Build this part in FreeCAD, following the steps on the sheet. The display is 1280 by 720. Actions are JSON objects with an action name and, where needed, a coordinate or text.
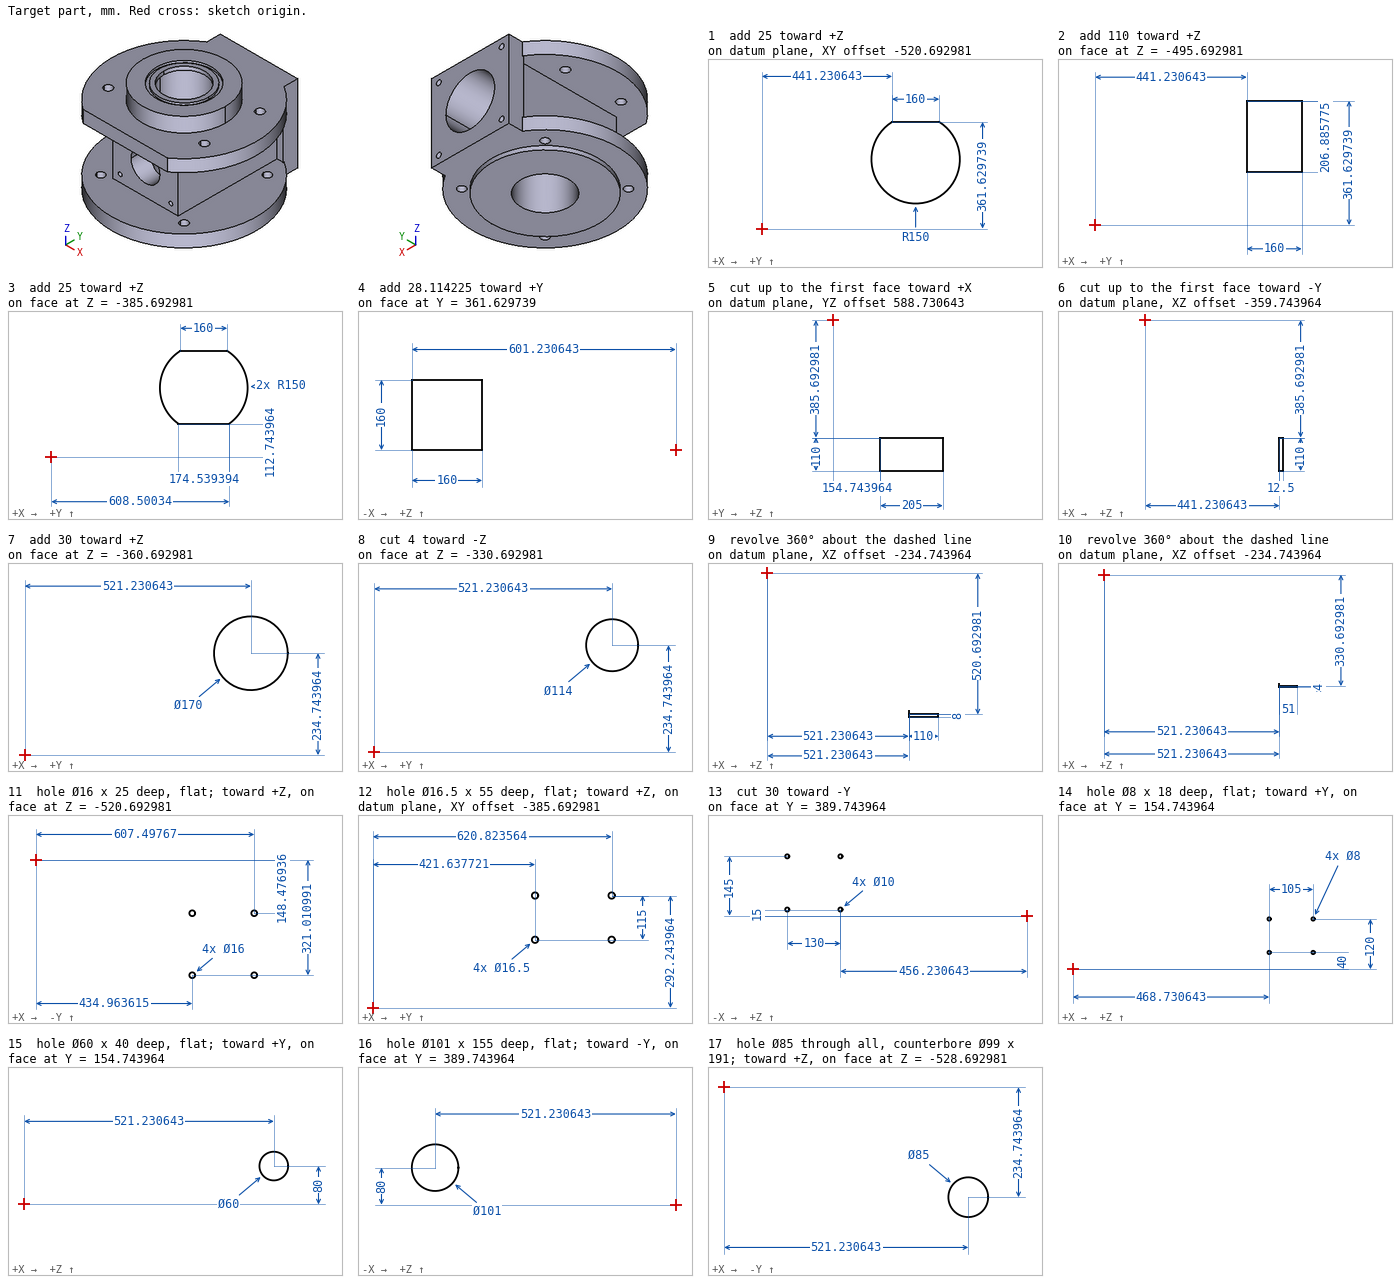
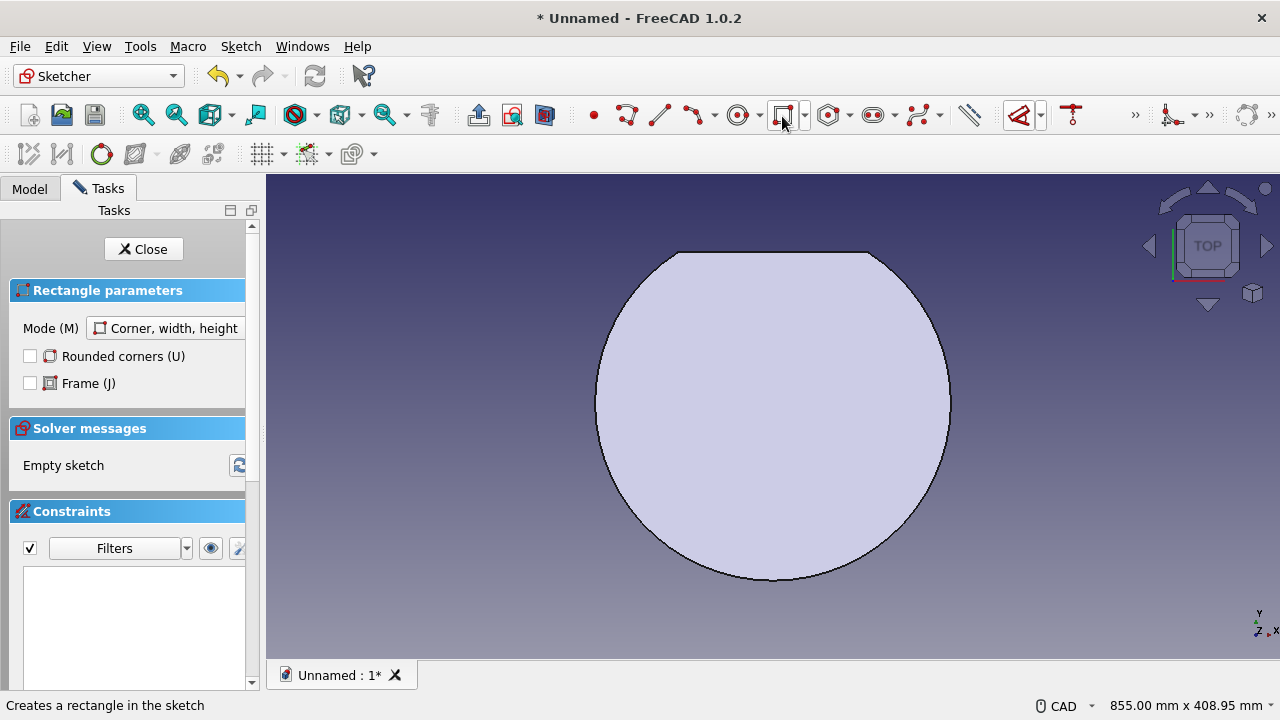
{"action": "left_click", "coordinate": [678, 252]}
{"action": "left_click", "coordinate": [868, 498]}
{"action": "key", "text": "Escape"}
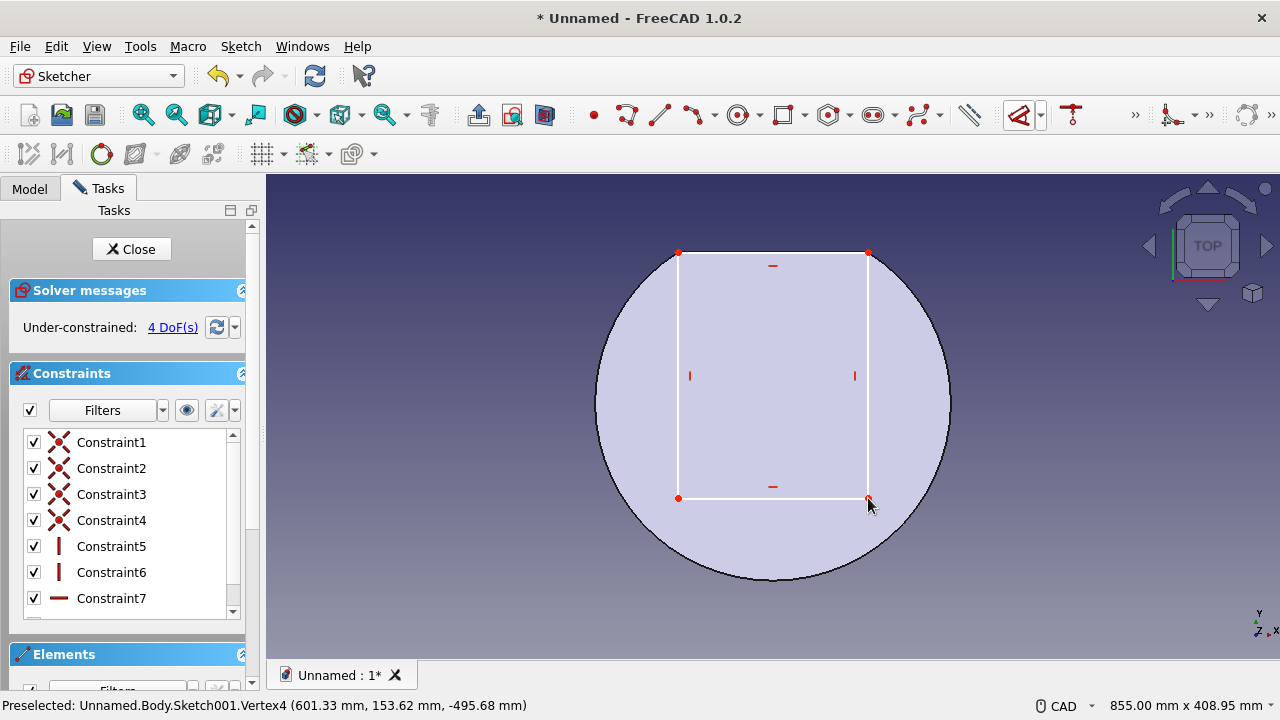
{"action": "left_click", "coordinate": [735, 499]}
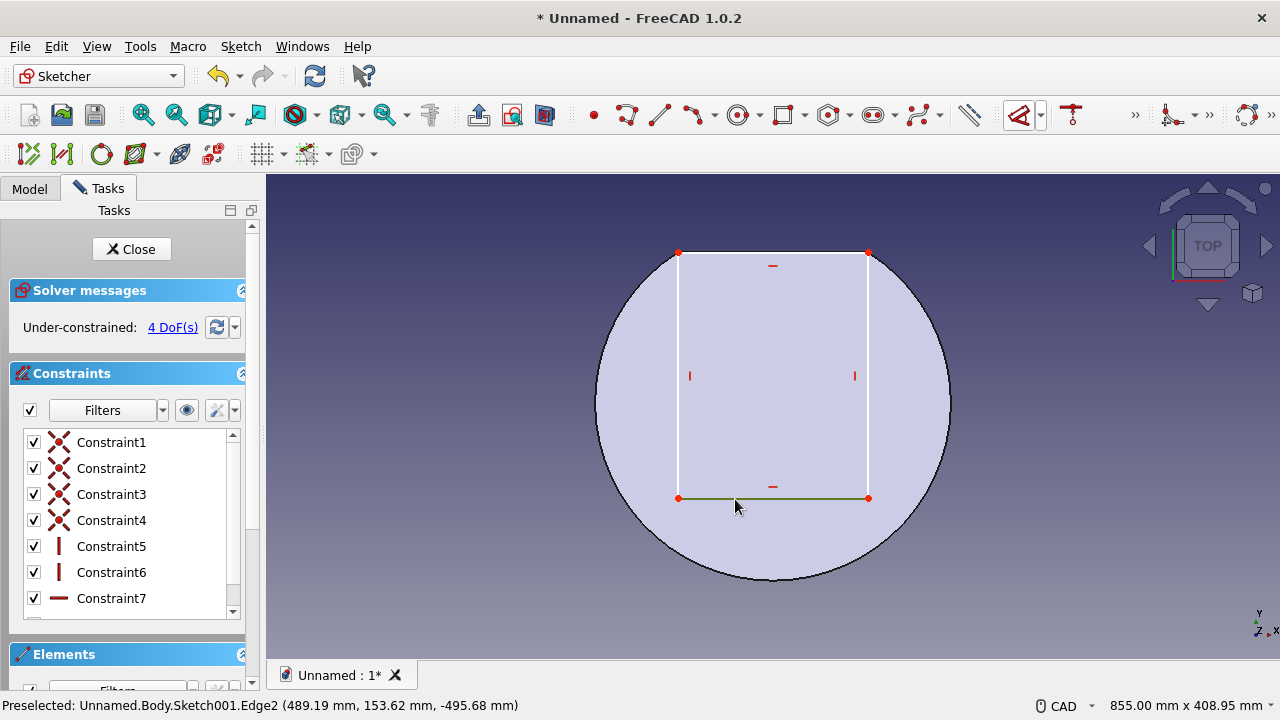
{"action": "left_click", "coordinate": [1040, 116]}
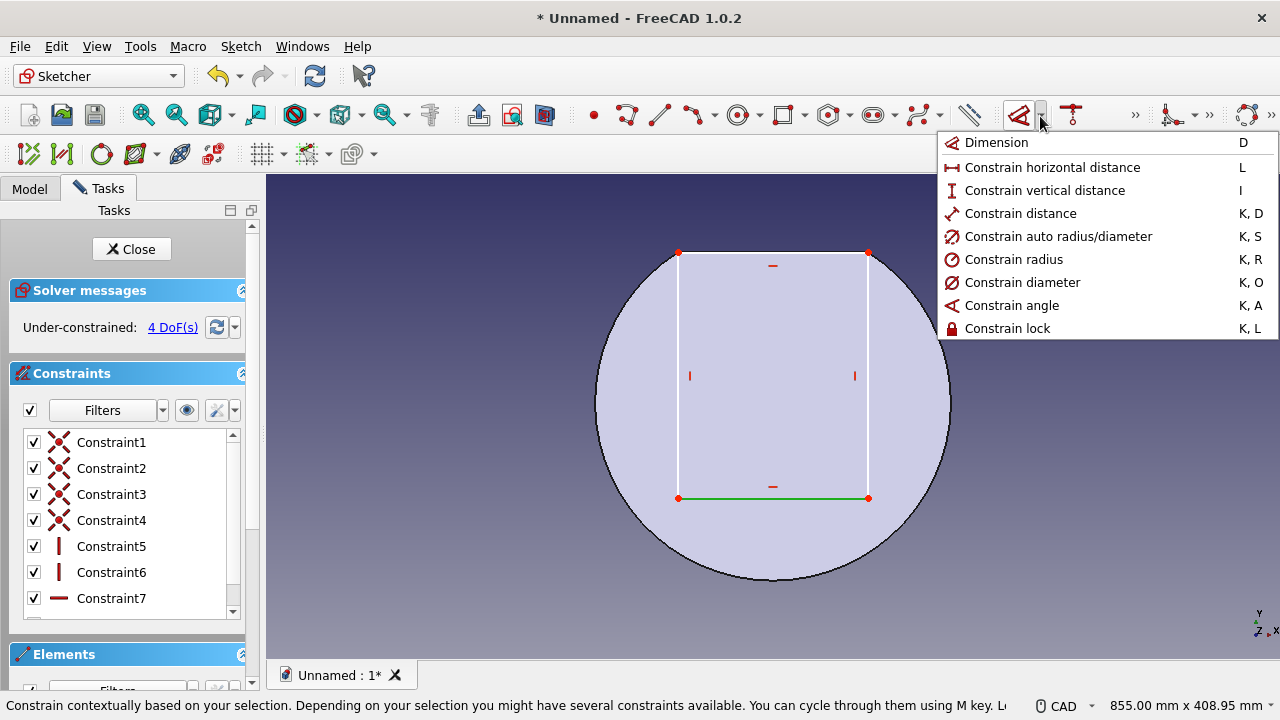
{"action": "left_click", "coordinate": [1108, 168]}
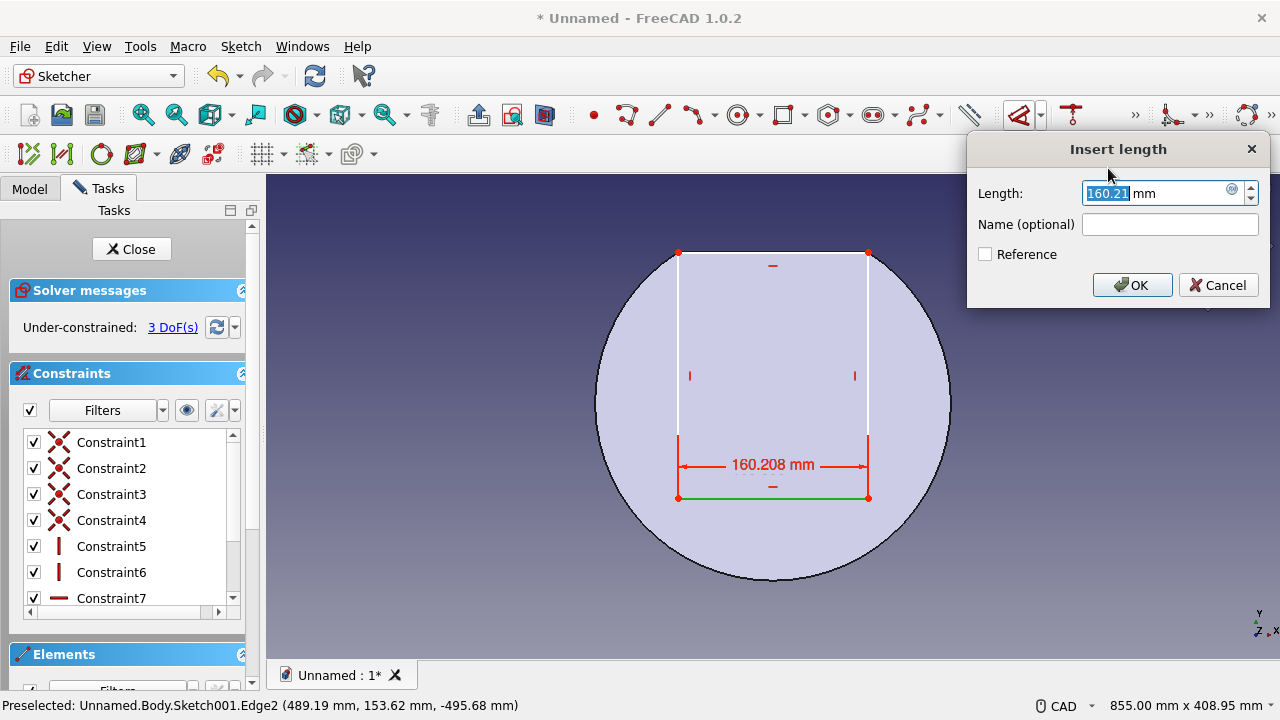
{"action": "type", "text": "160"}
{"action": "key", "text": "Return"}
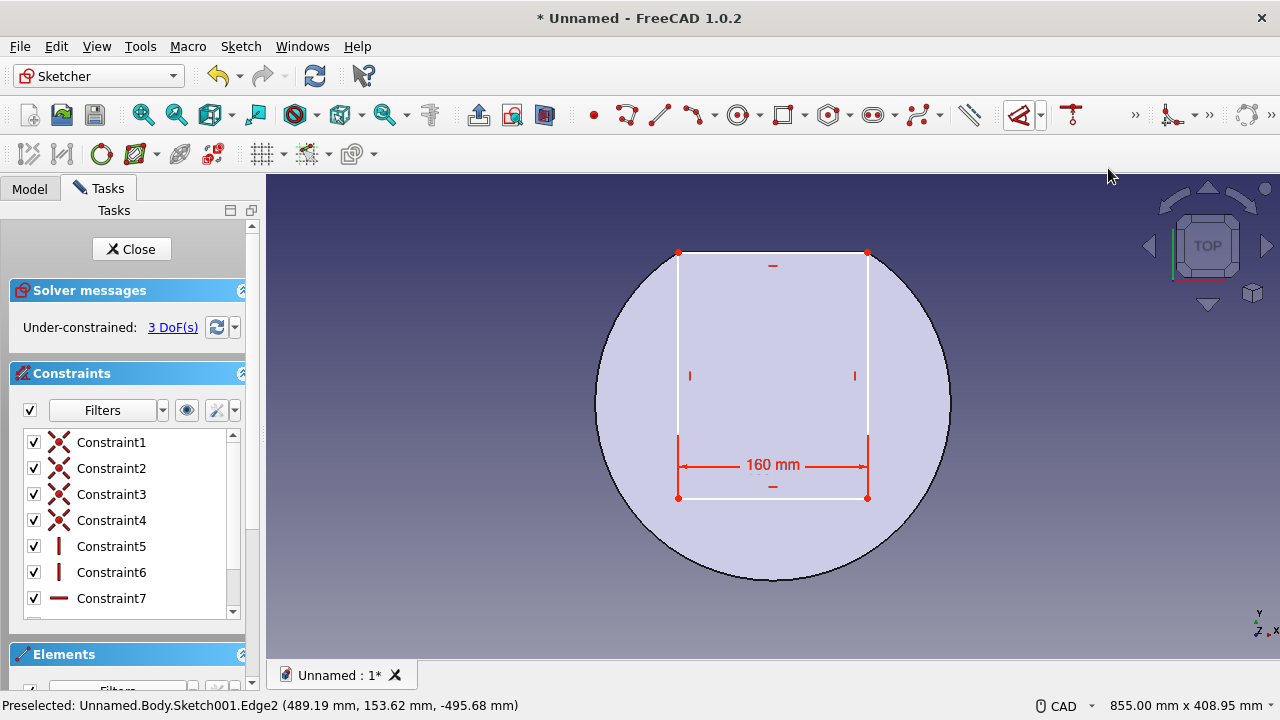
{"action": "left_click", "coordinate": [678, 327]}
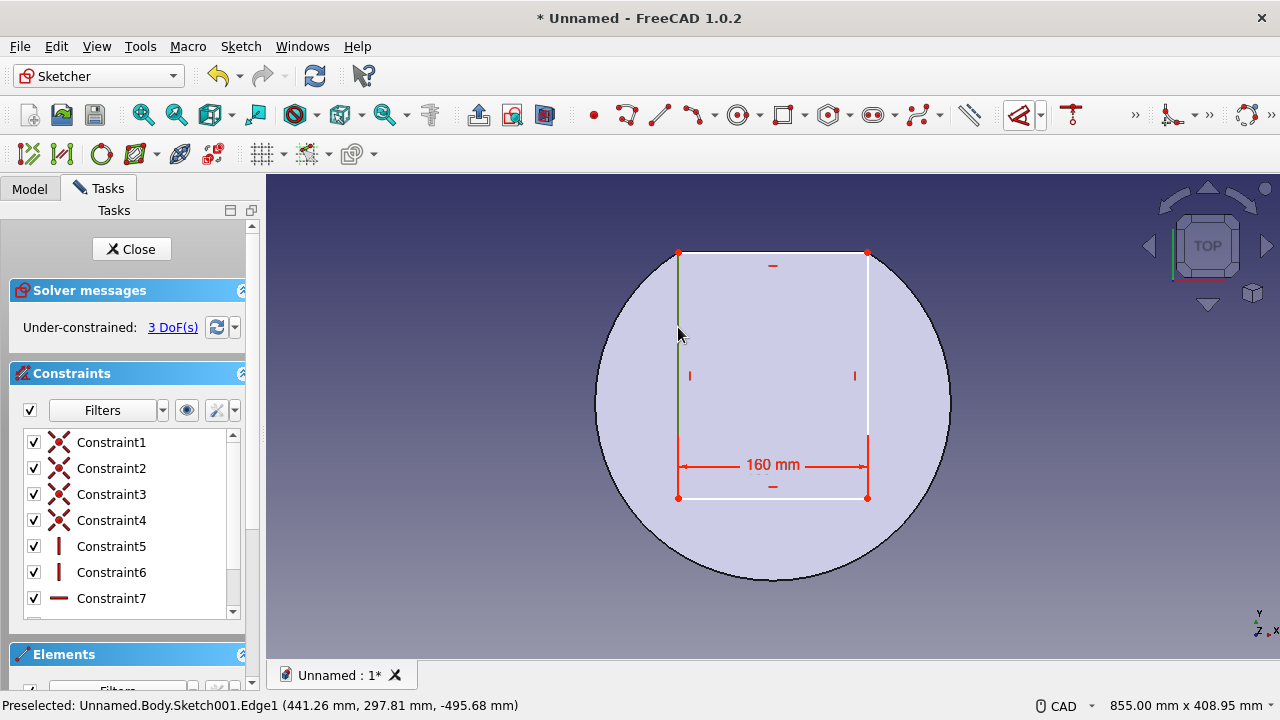
{"action": "left_click", "coordinate": [1040, 116]}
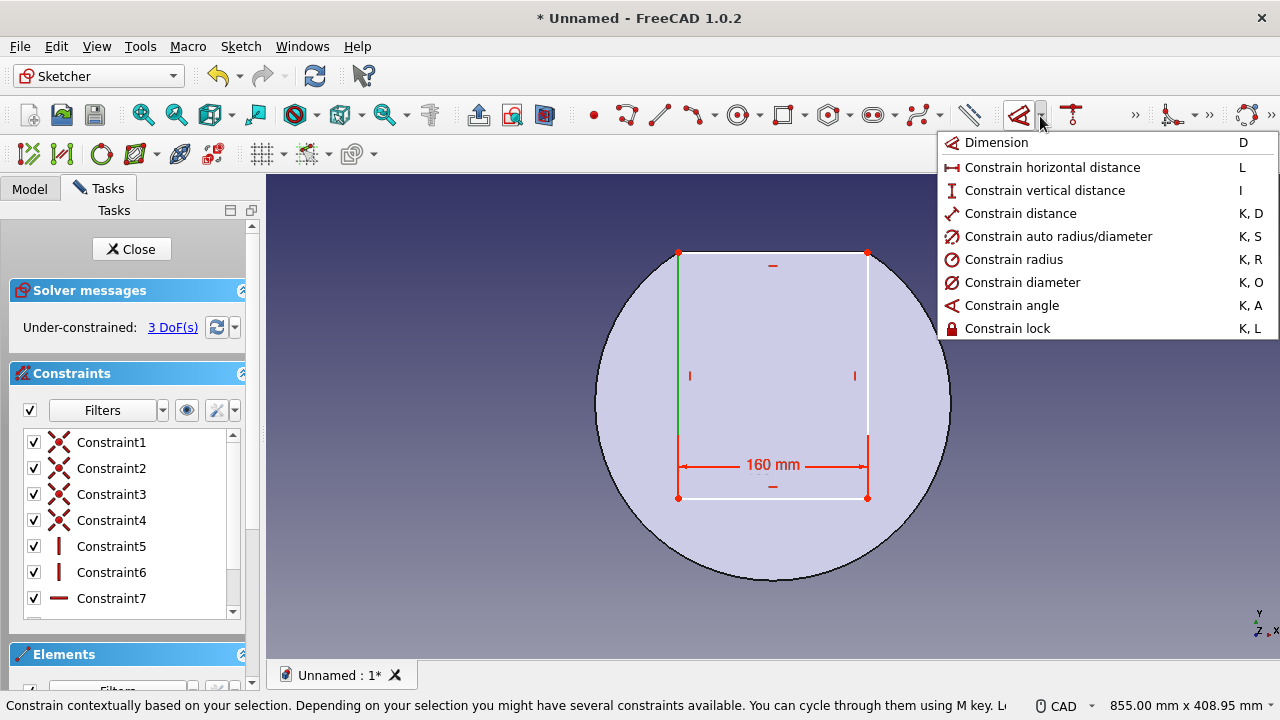
{"action": "left_click", "coordinate": [1108, 190]}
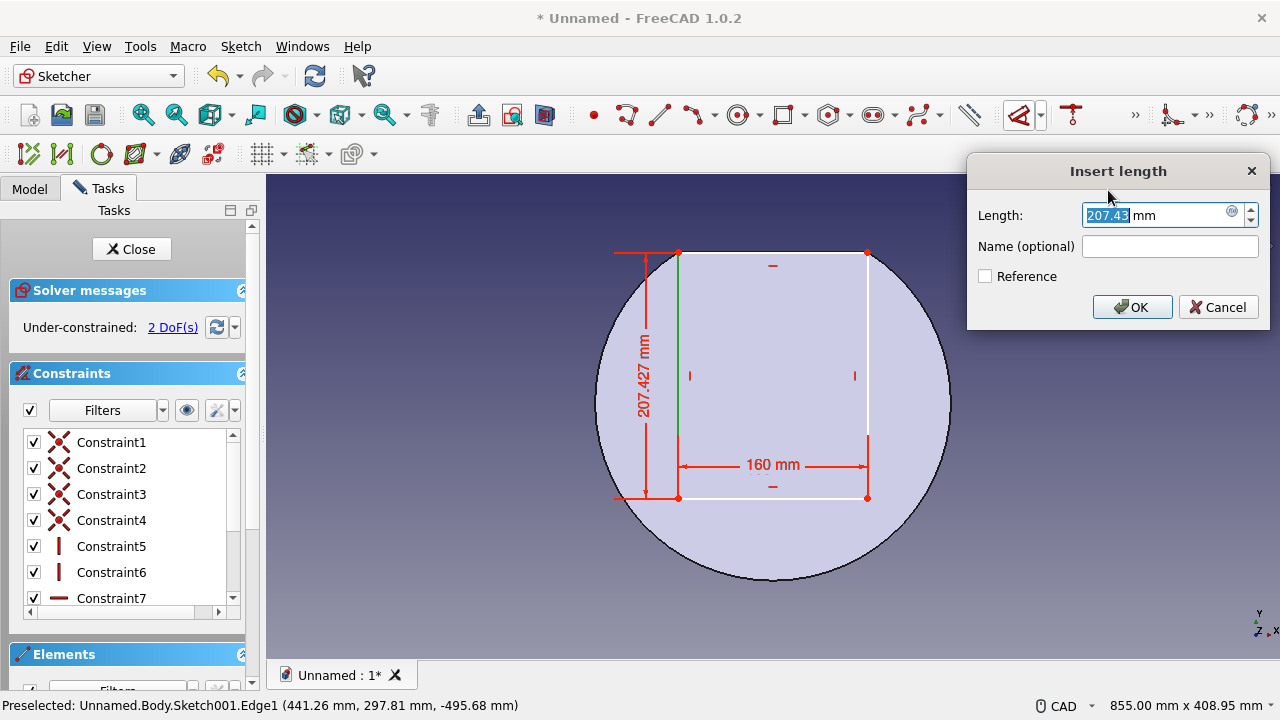
{"action": "type", "text": "206.885775"}
{"action": "key", "text": "Return"}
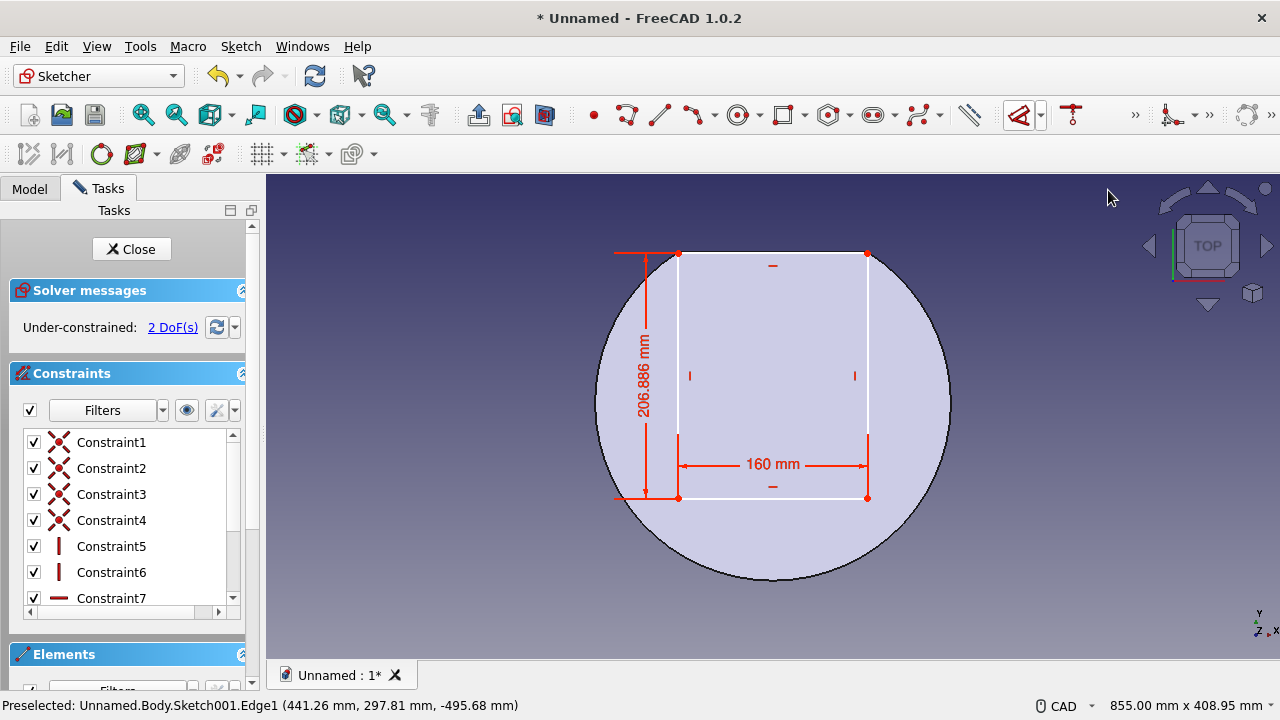
{"action": "left_click", "coordinate": [678, 253]}